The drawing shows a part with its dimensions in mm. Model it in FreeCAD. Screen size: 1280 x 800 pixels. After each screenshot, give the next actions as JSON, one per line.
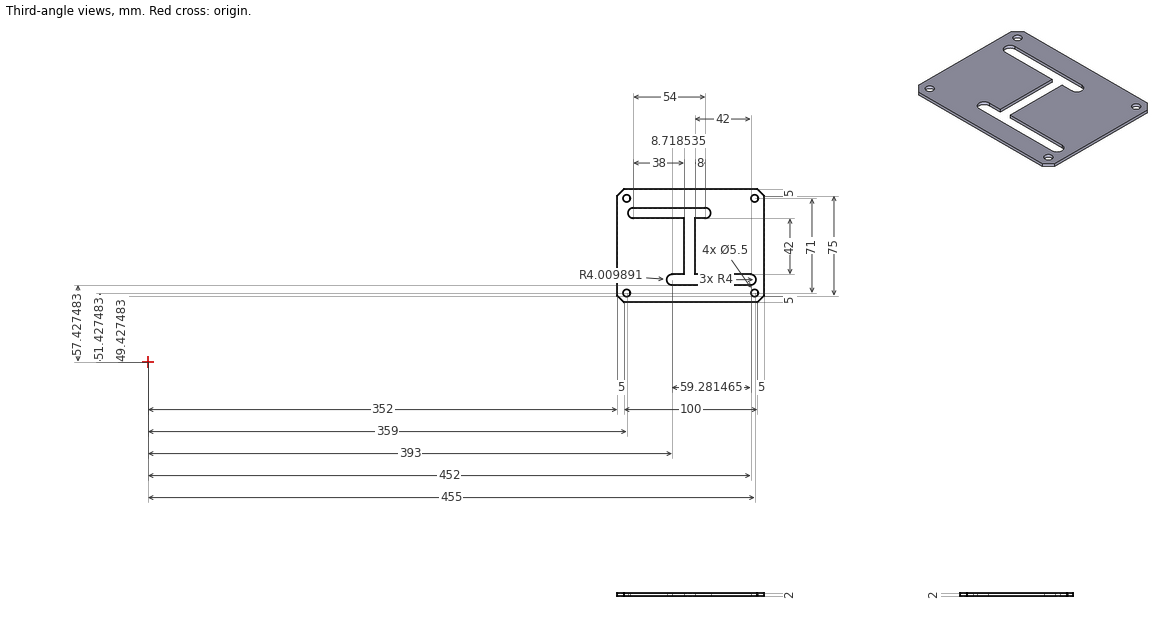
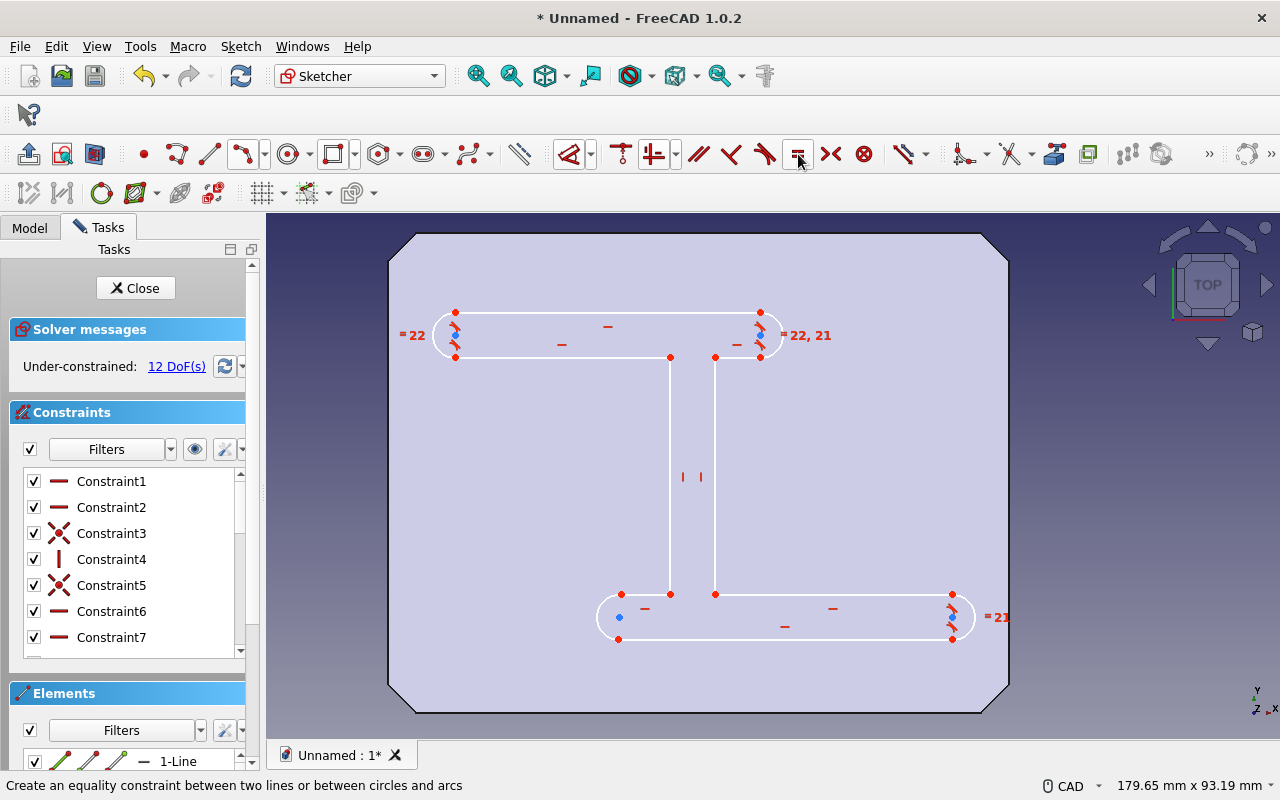
{"action": "scroll", "coordinate": [971, 631], "scroll_direction": "up", "scroll_amount": 3}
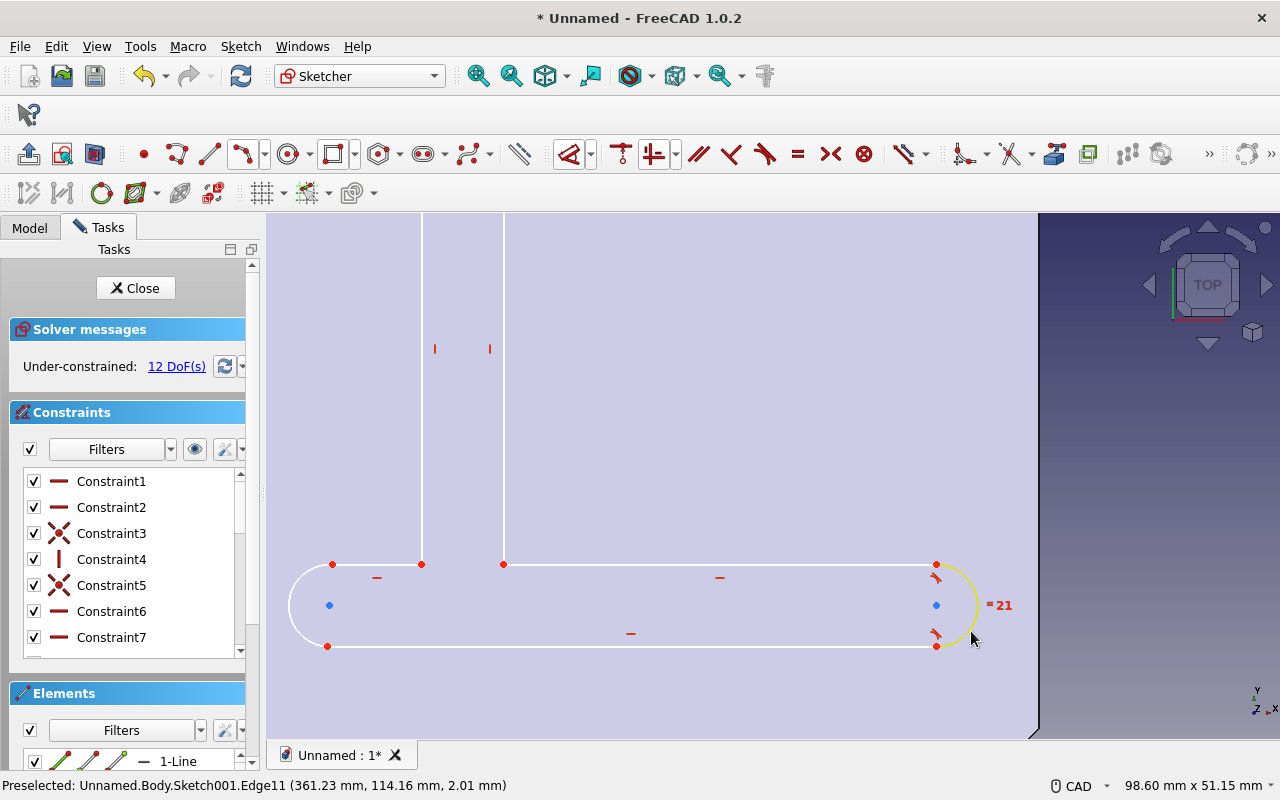
{"action": "left_click", "coordinate": [970, 630]}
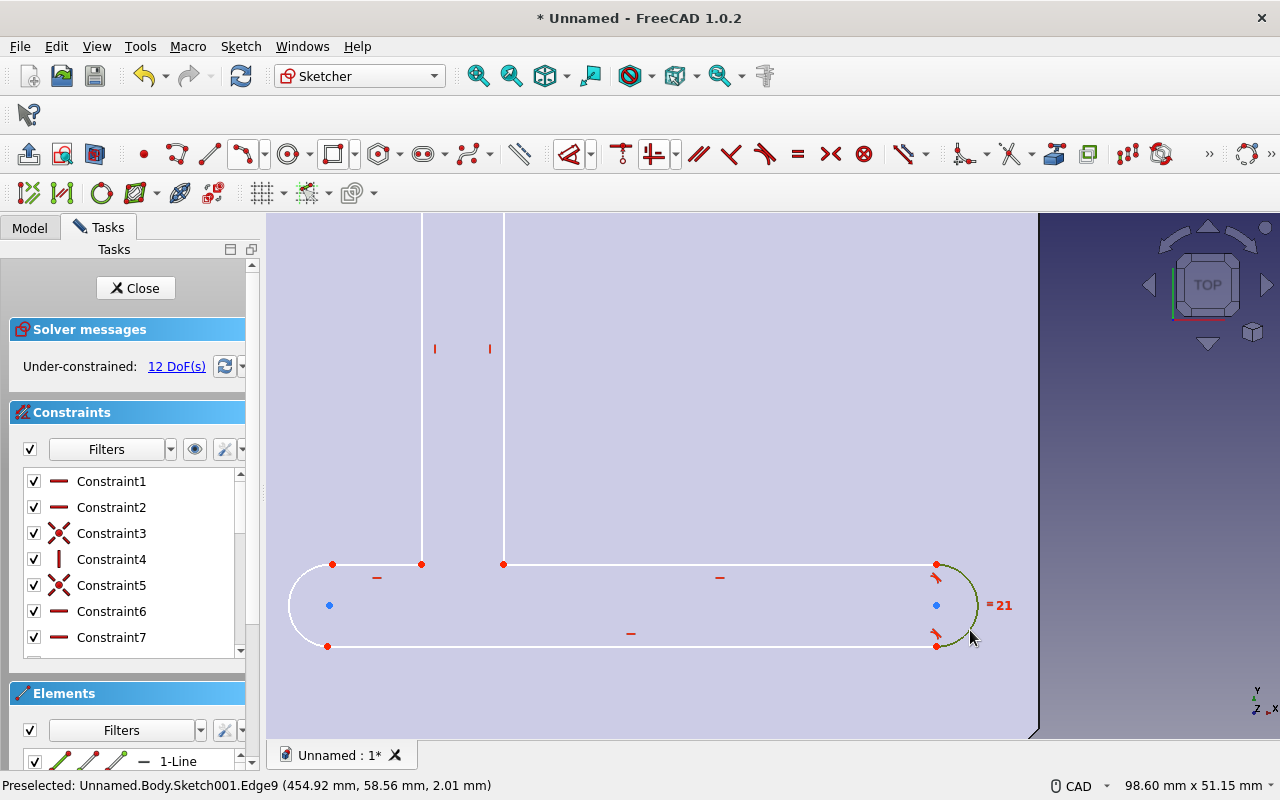
{"action": "left_click", "coordinate": [590, 154]}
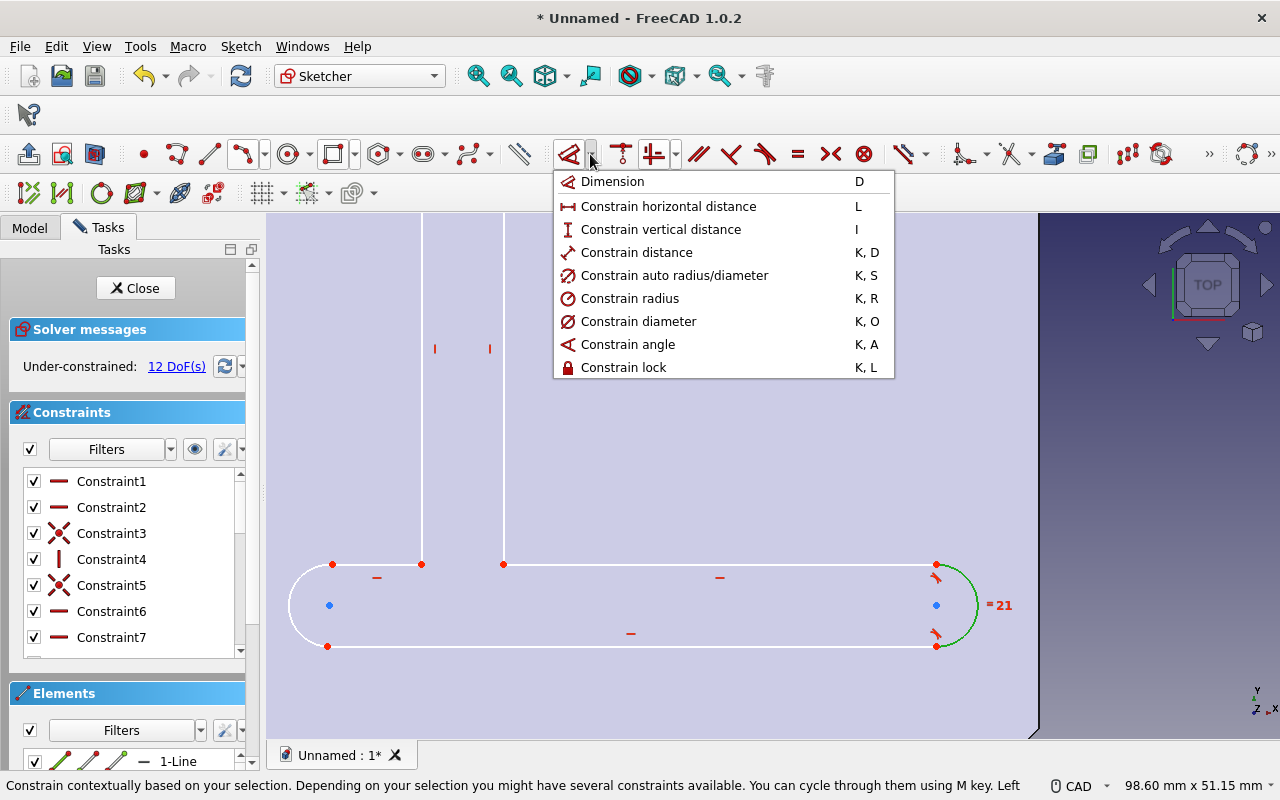
{"action": "left_click", "coordinate": [724, 298]}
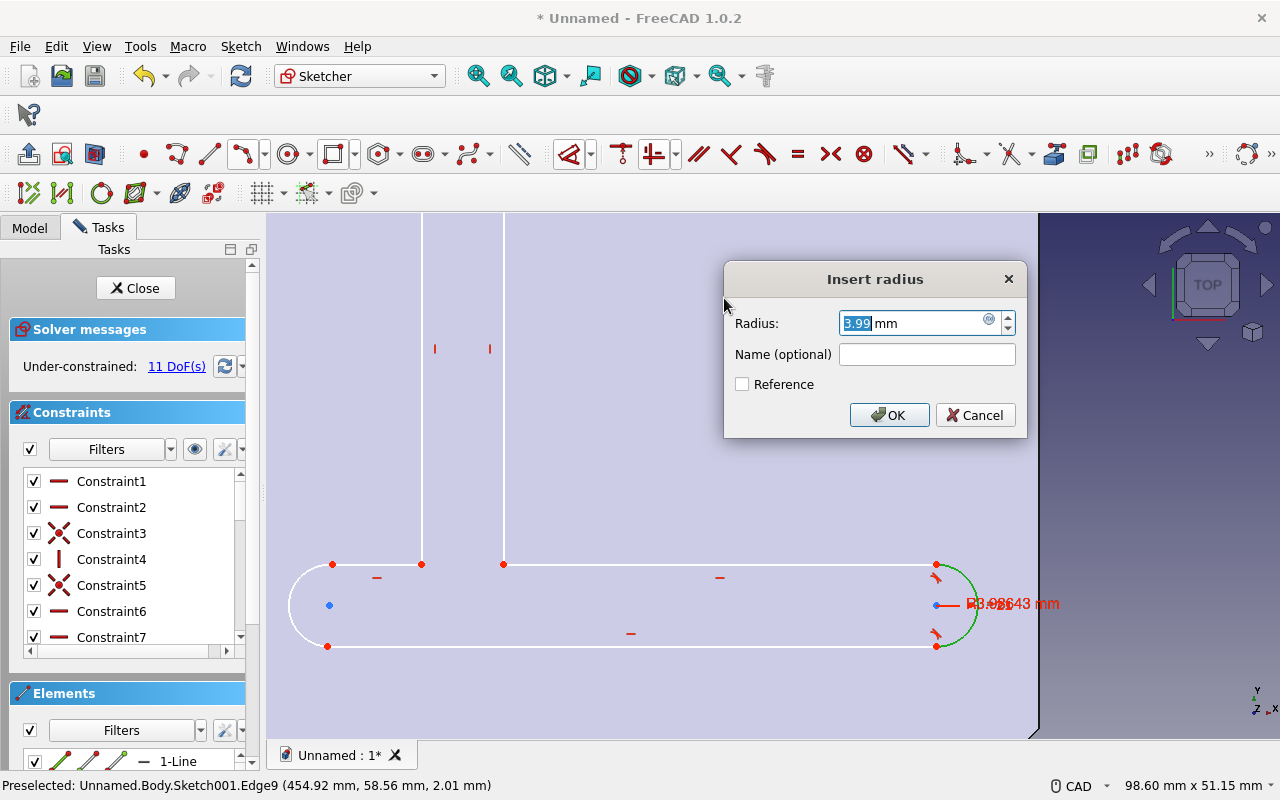
{"action": "type", "text": "4"}
{"action": "key", "text": "Return"}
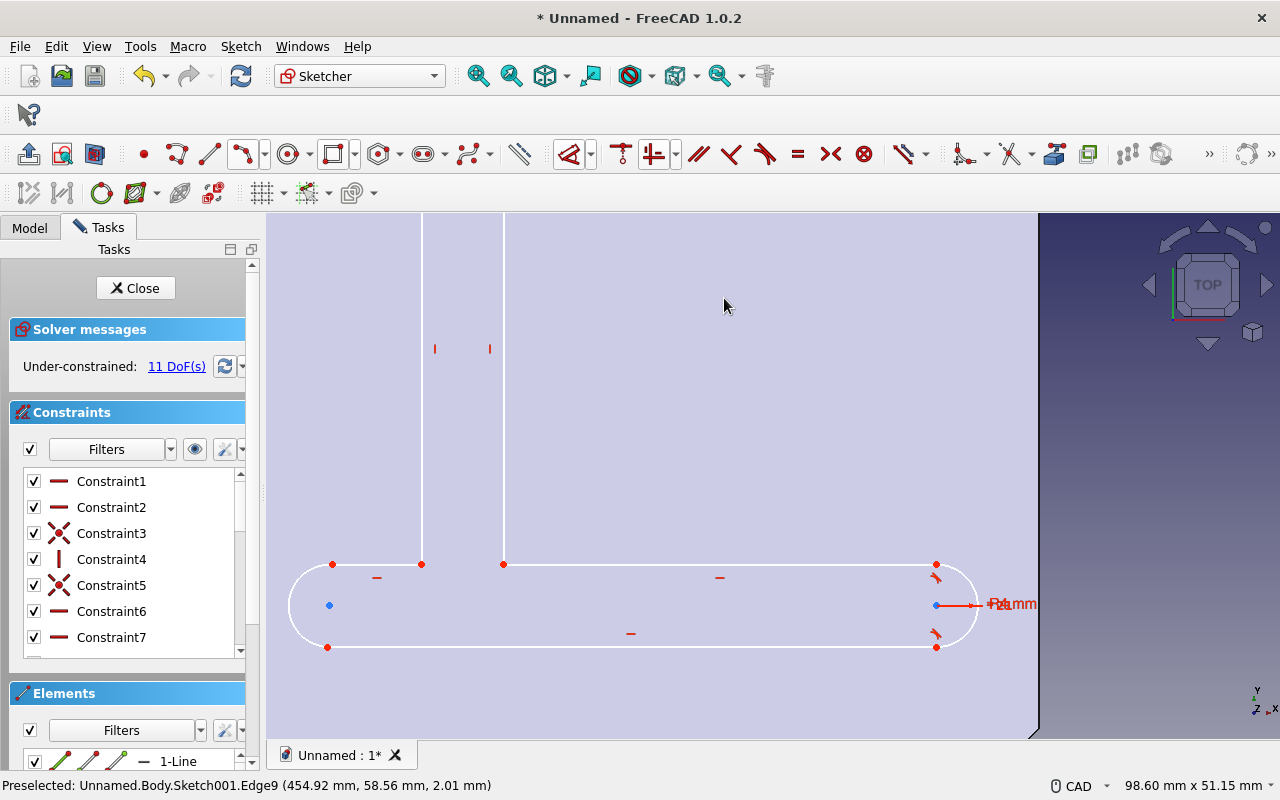
{"action": "left_click", "coordinate": [298, 579]}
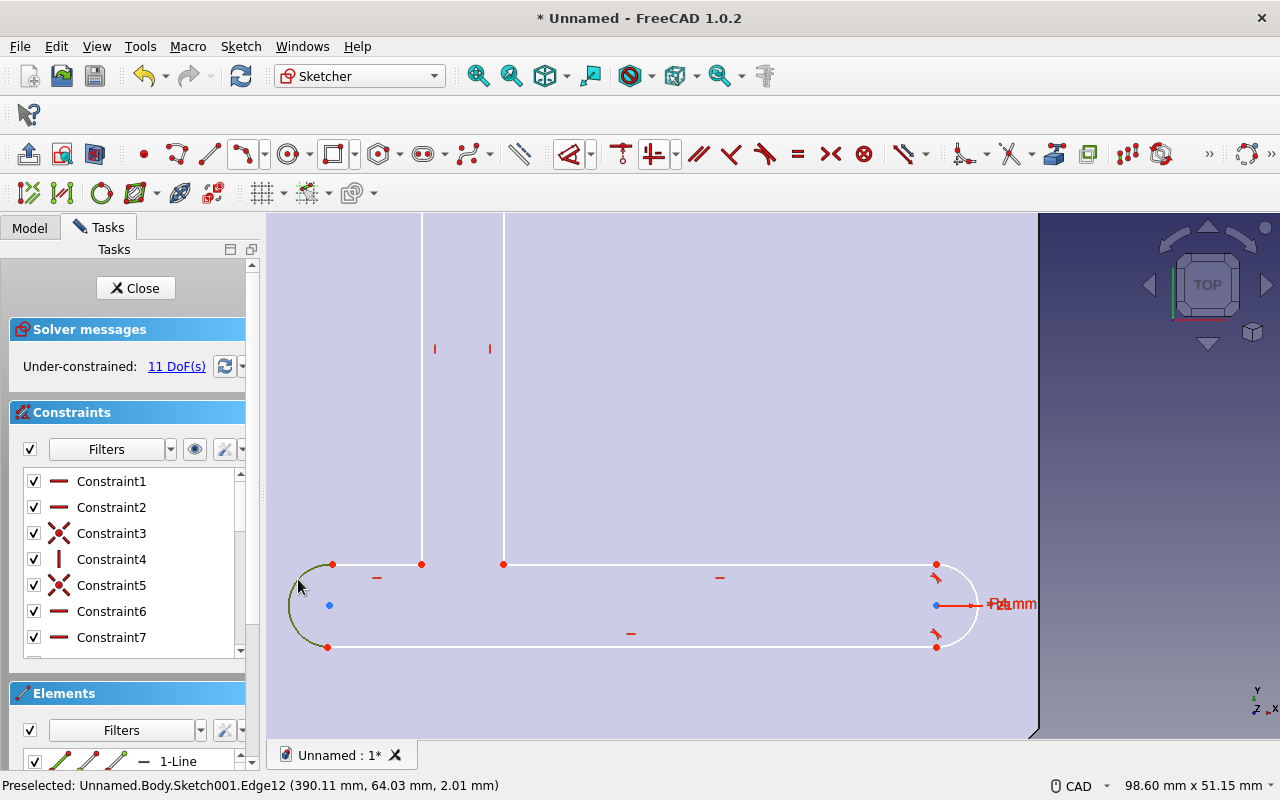
{"action": "key", "text": "k r"}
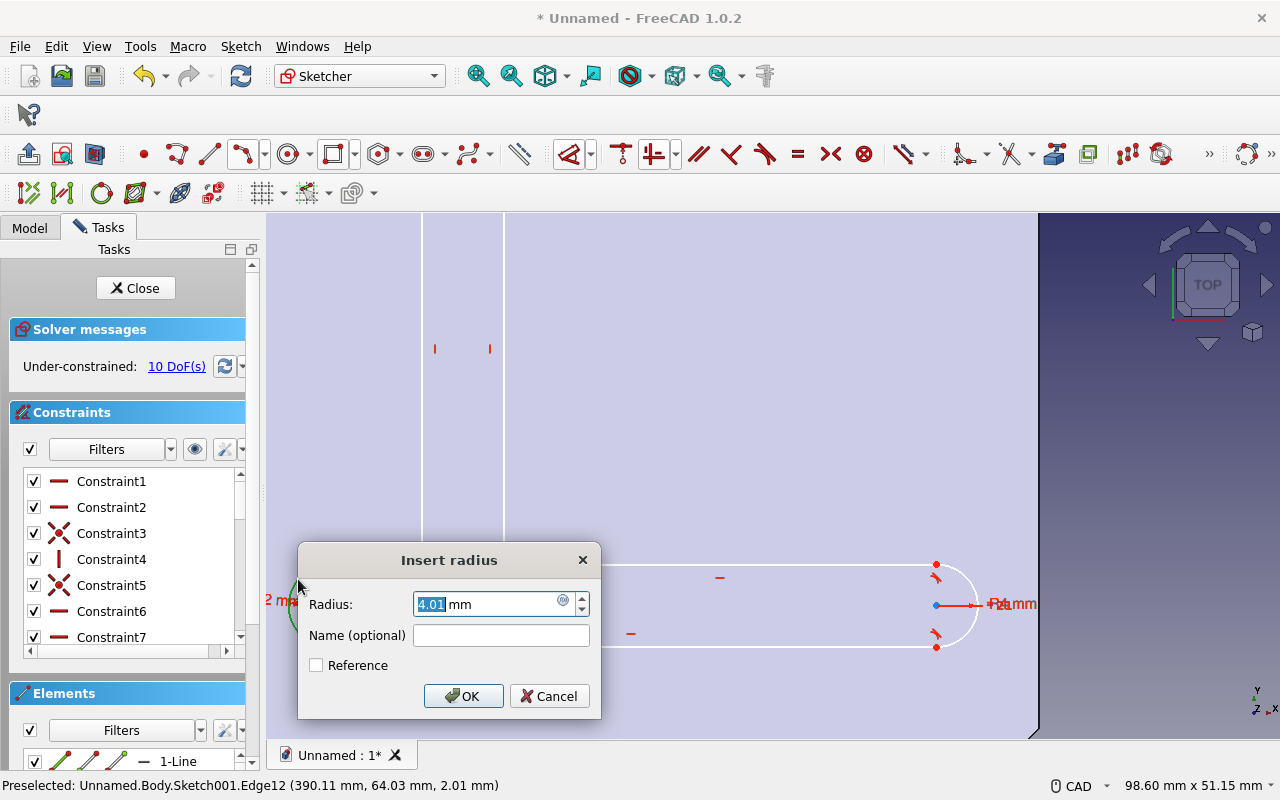
{"action": "type", "text": "4.009891"}
{"action": "key", "text": "Return"}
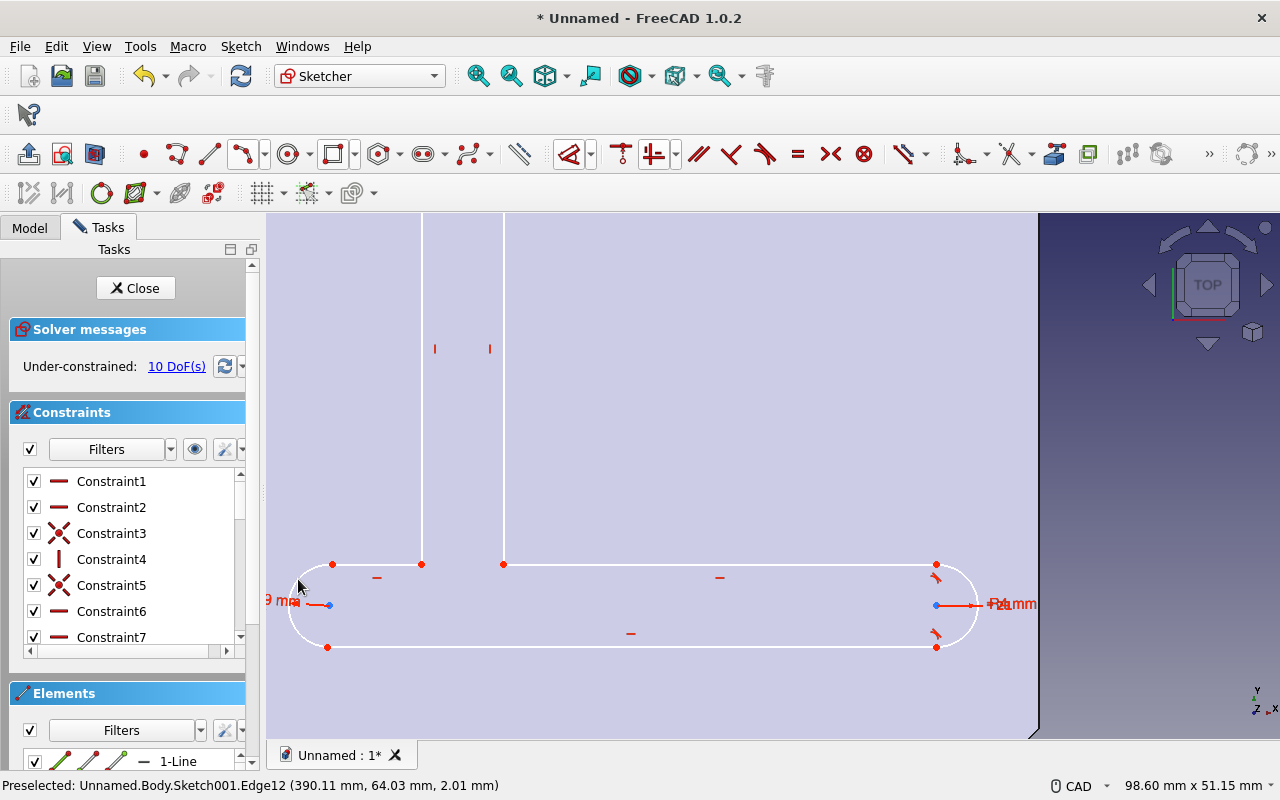
{"action": "scroll", "coordinate": [973, 633], "scroll_direction": "down", "scroll_amount": 3}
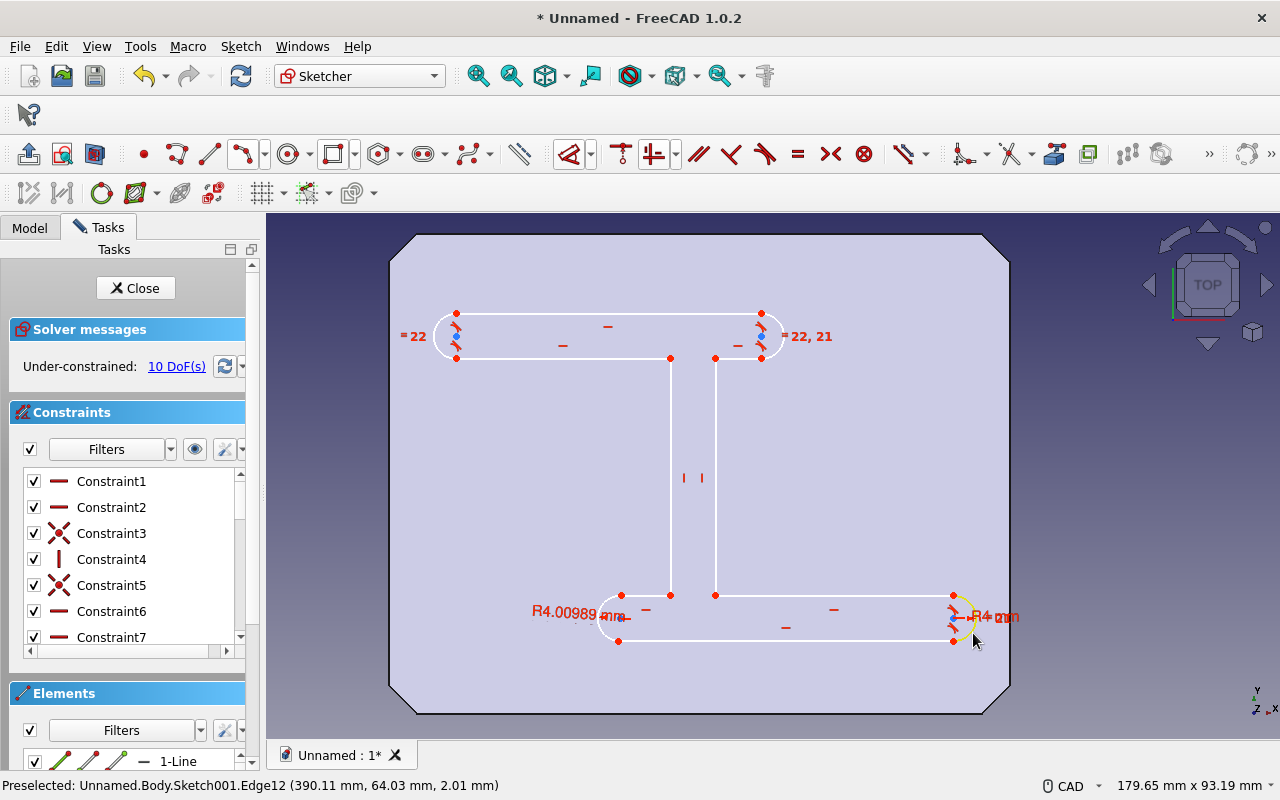
{"action": "left_click", "coordinate": [730, 359]}